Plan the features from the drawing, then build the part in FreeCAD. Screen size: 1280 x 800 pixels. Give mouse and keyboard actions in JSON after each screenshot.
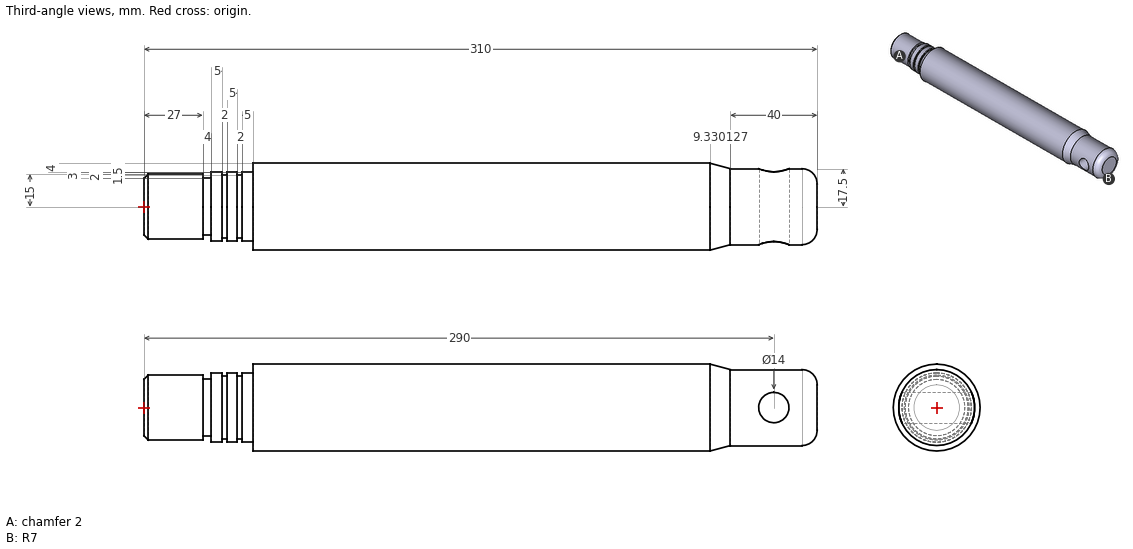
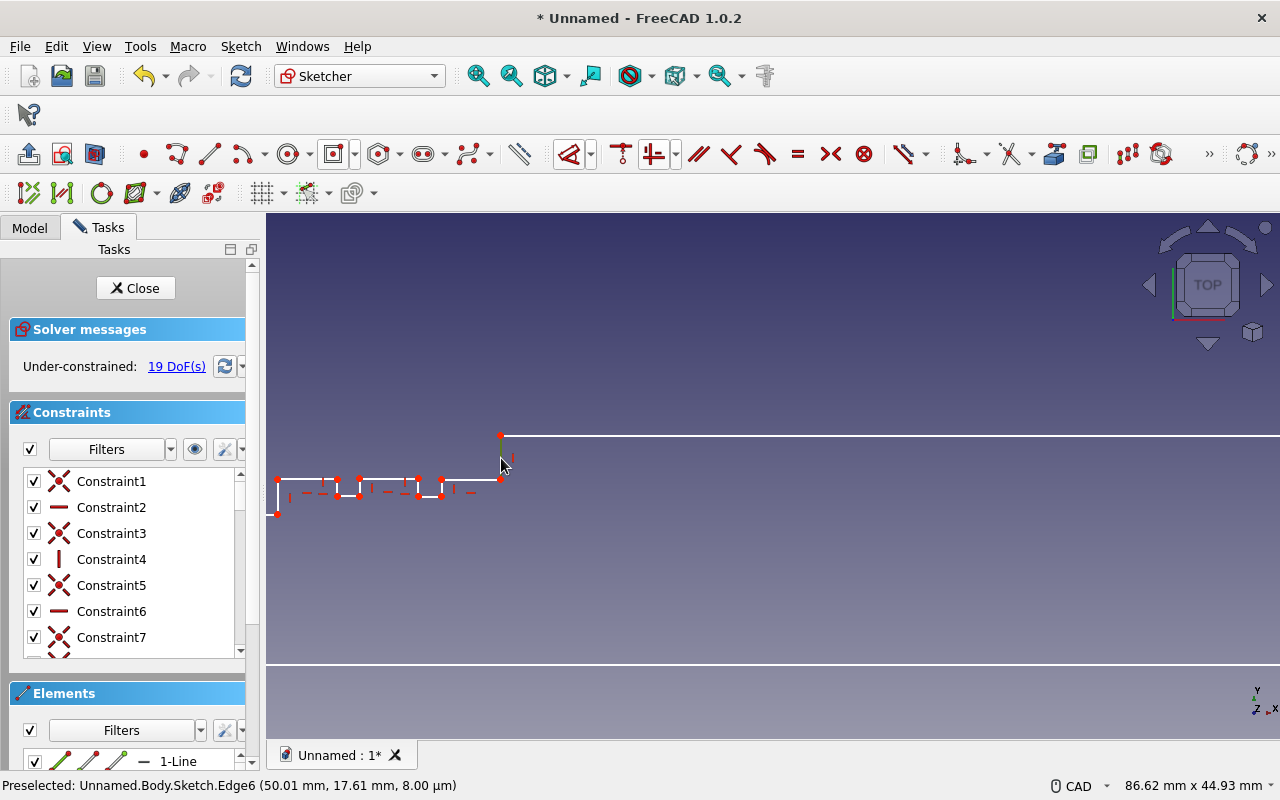
{"action": "left_click", "coordinate": [590, 154]}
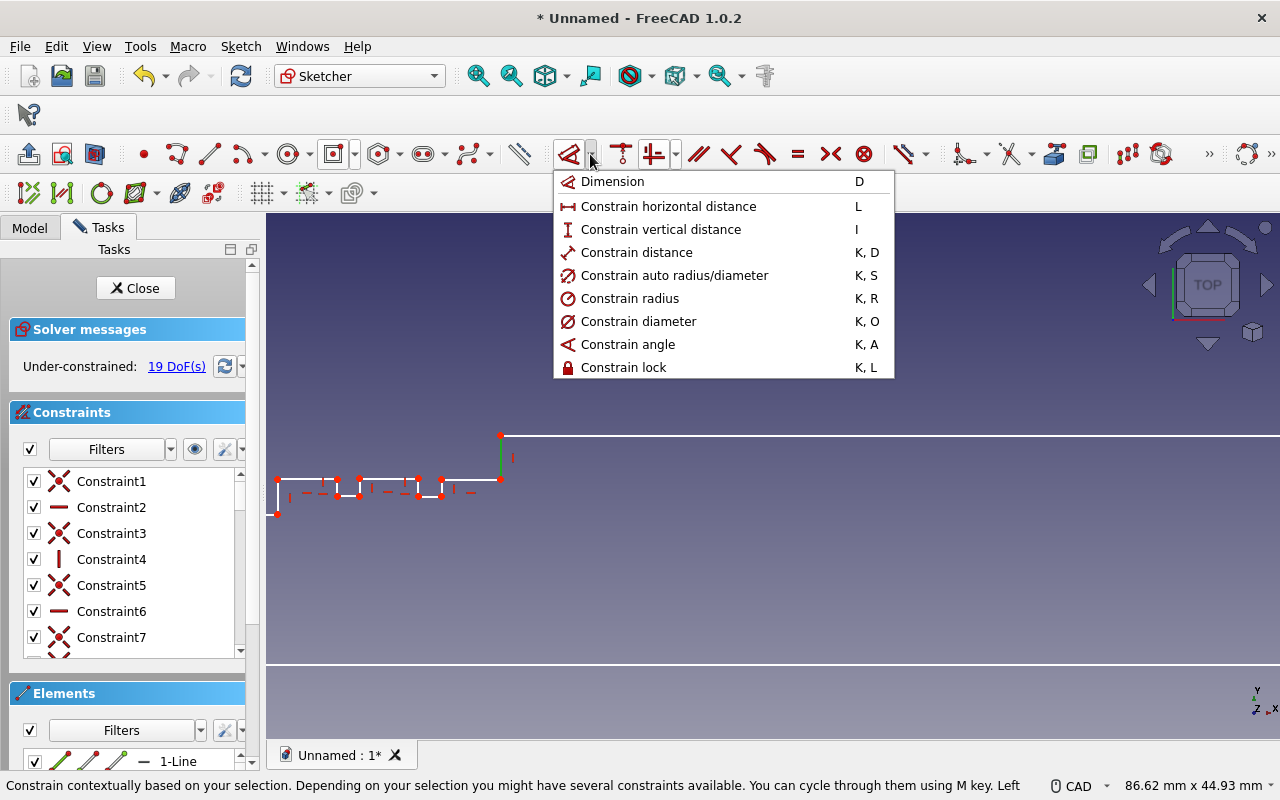
{"action": "left_click", "coordinate": [724, 230]}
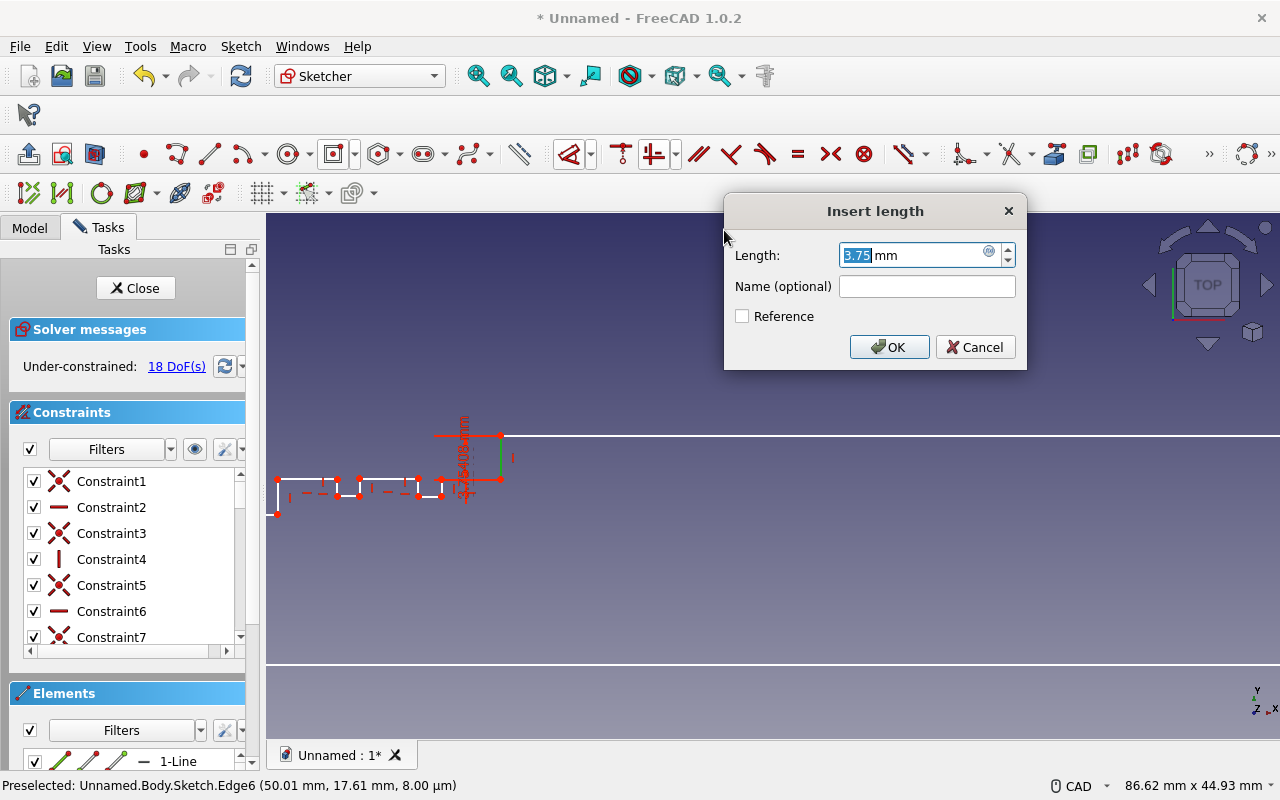
{"action": "type", "text": "4"}
{"action": "key", "text": "Return"}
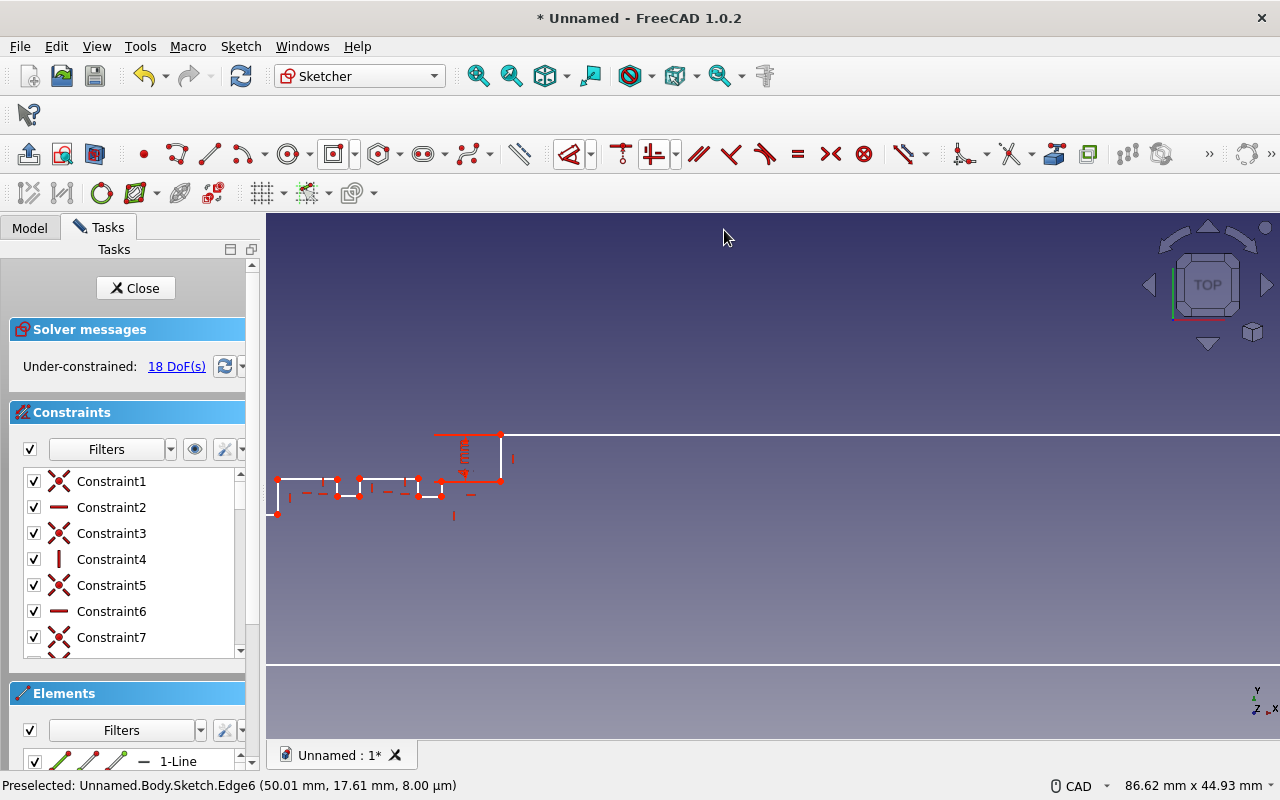
{"action": "left_click", "coordinate": [483, 482]}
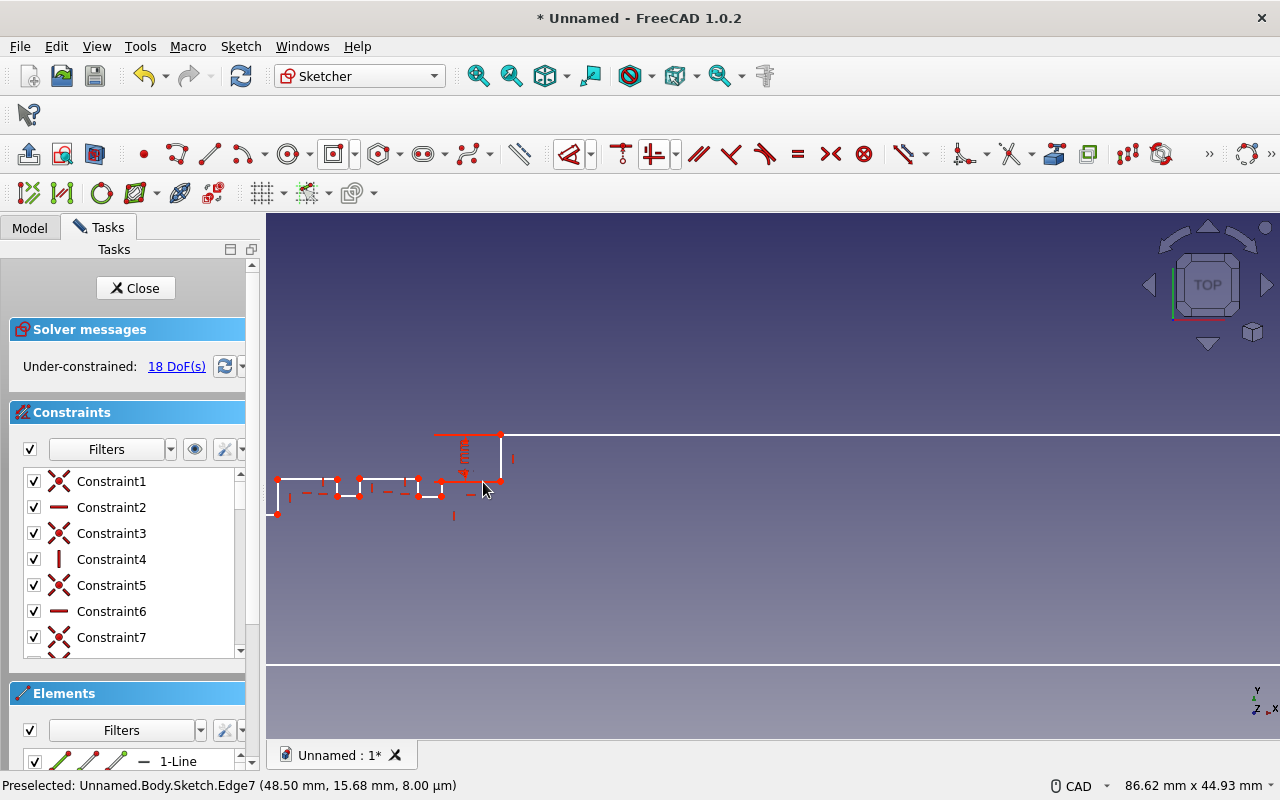
{"action": "key", "text": "l"}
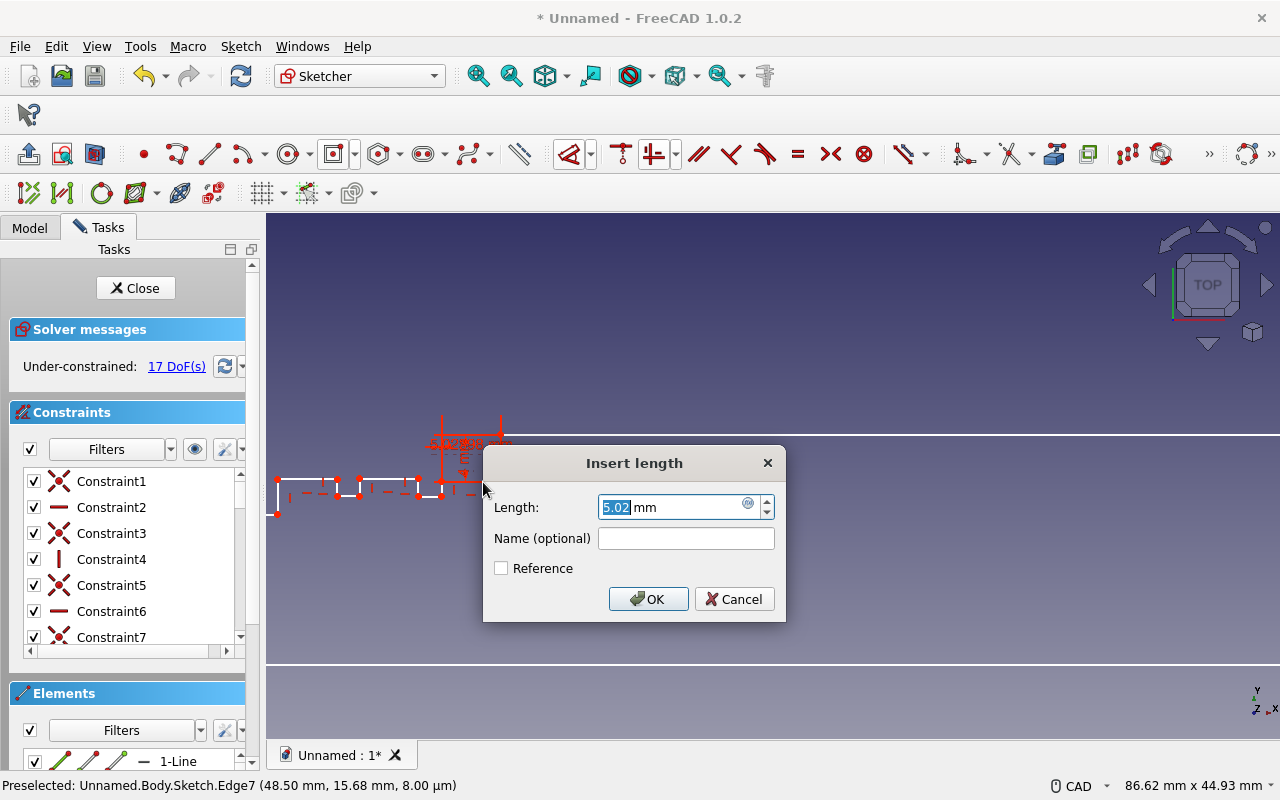
{"action": "type", "text": "5"}
{"action": "key", "text": "Return"}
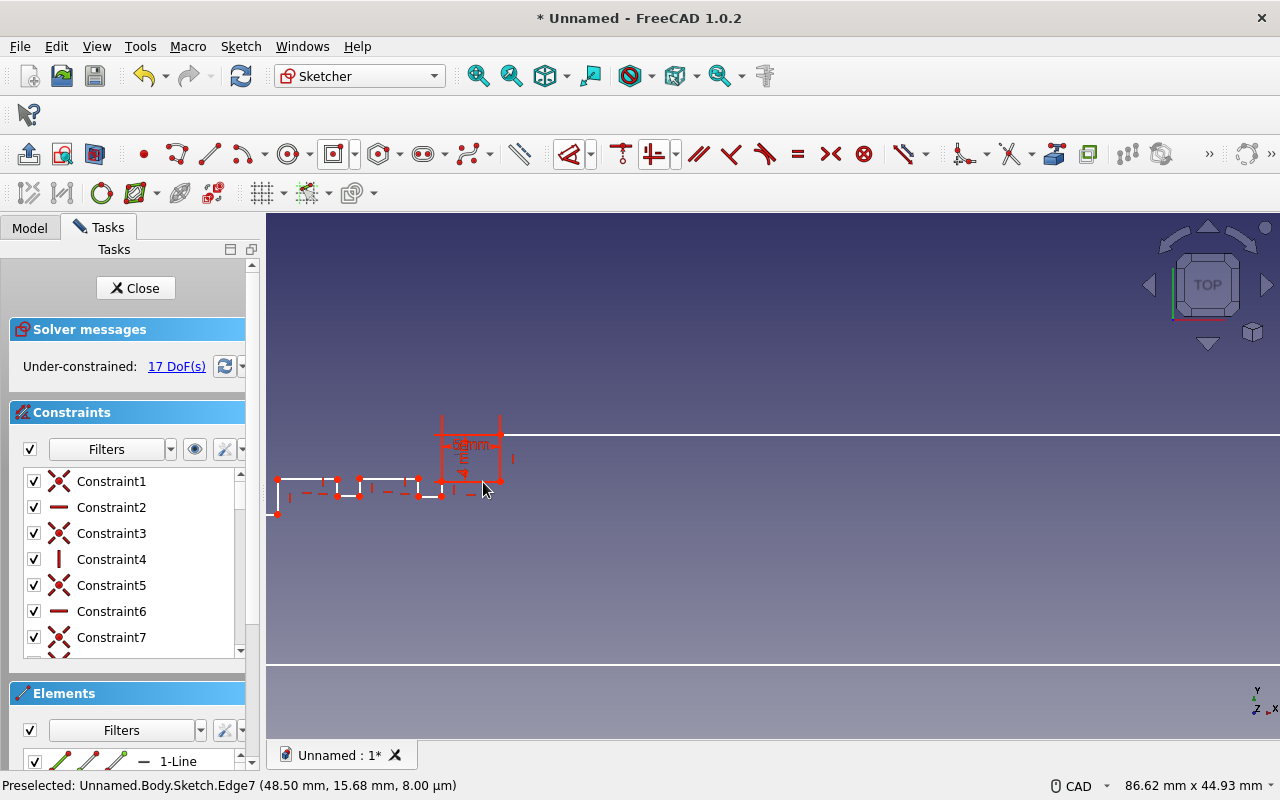
{"action": "scroll", "coordinate": [432, 497], "scroll_direction": "up", "scroll_amount": 3}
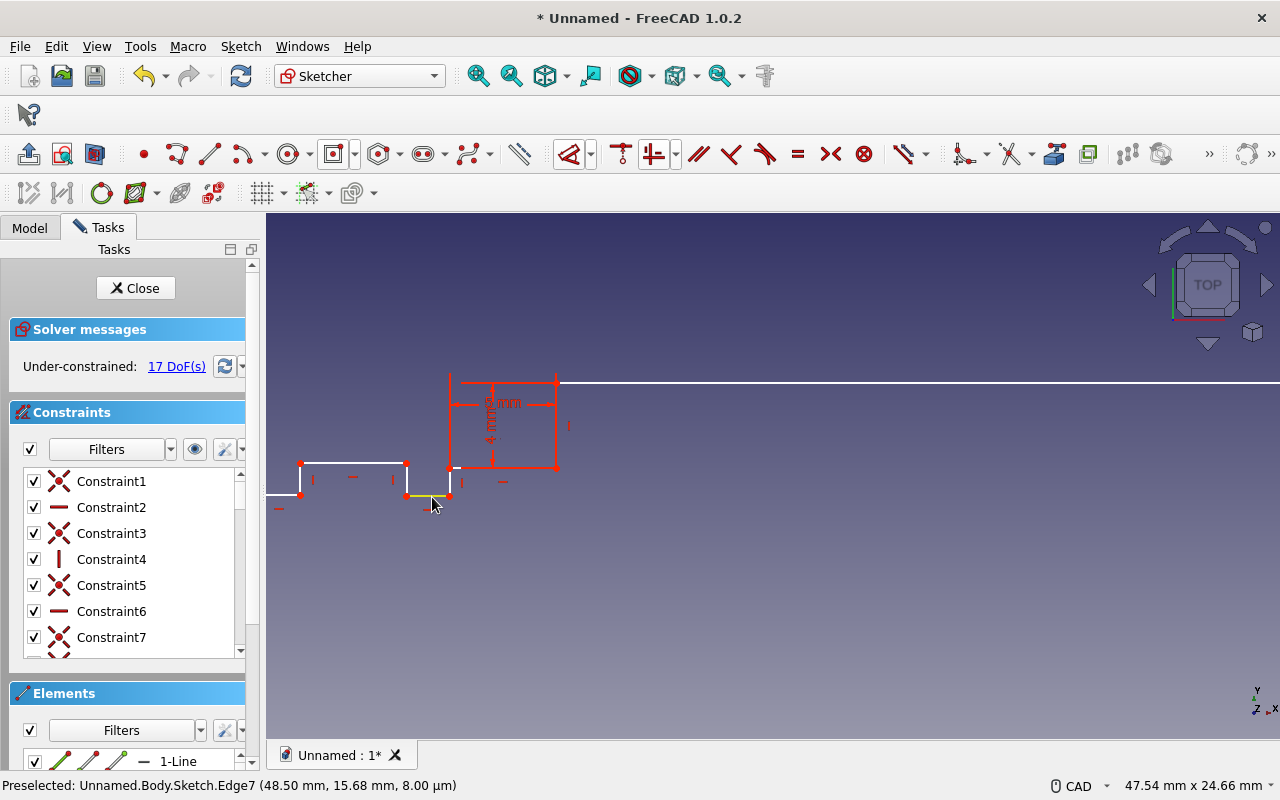
{"action": "left_click", "coordinate": [433, 496]}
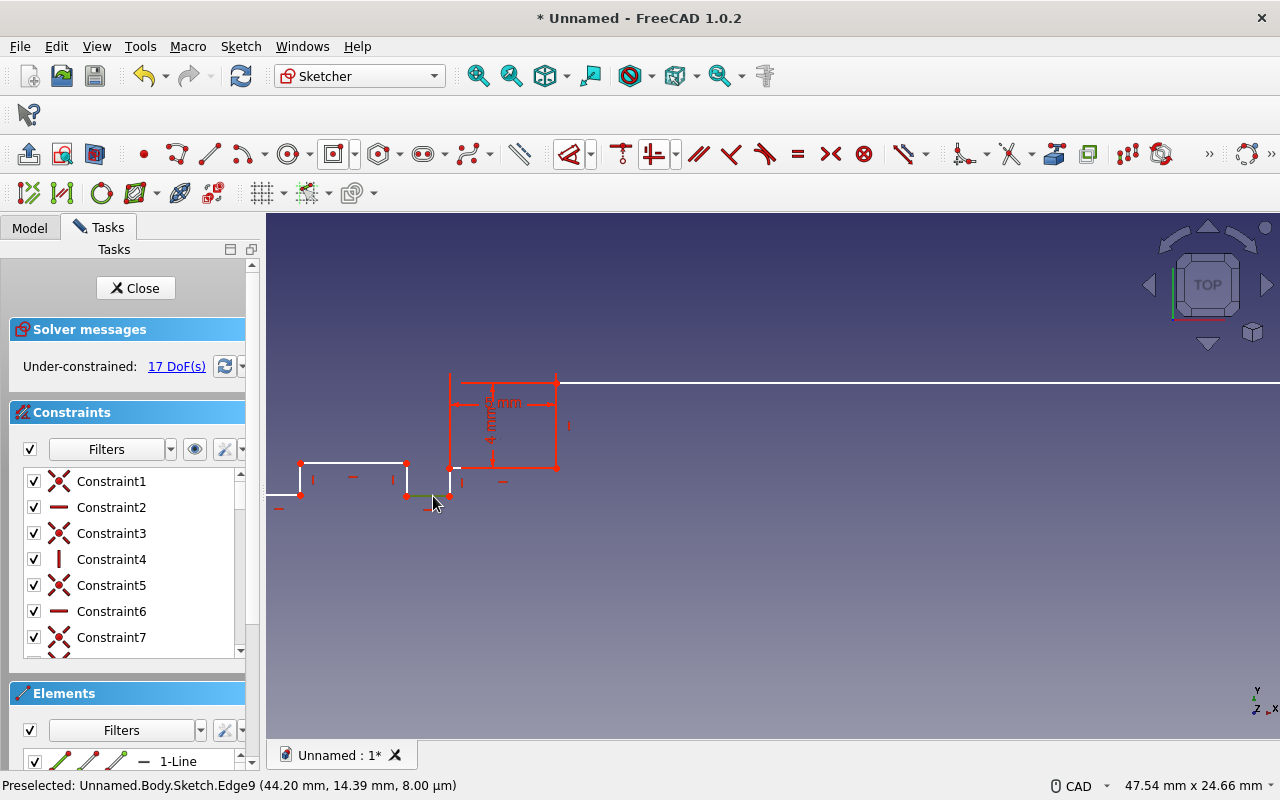
{"action": "left_click", "coordinate": [590, 154]}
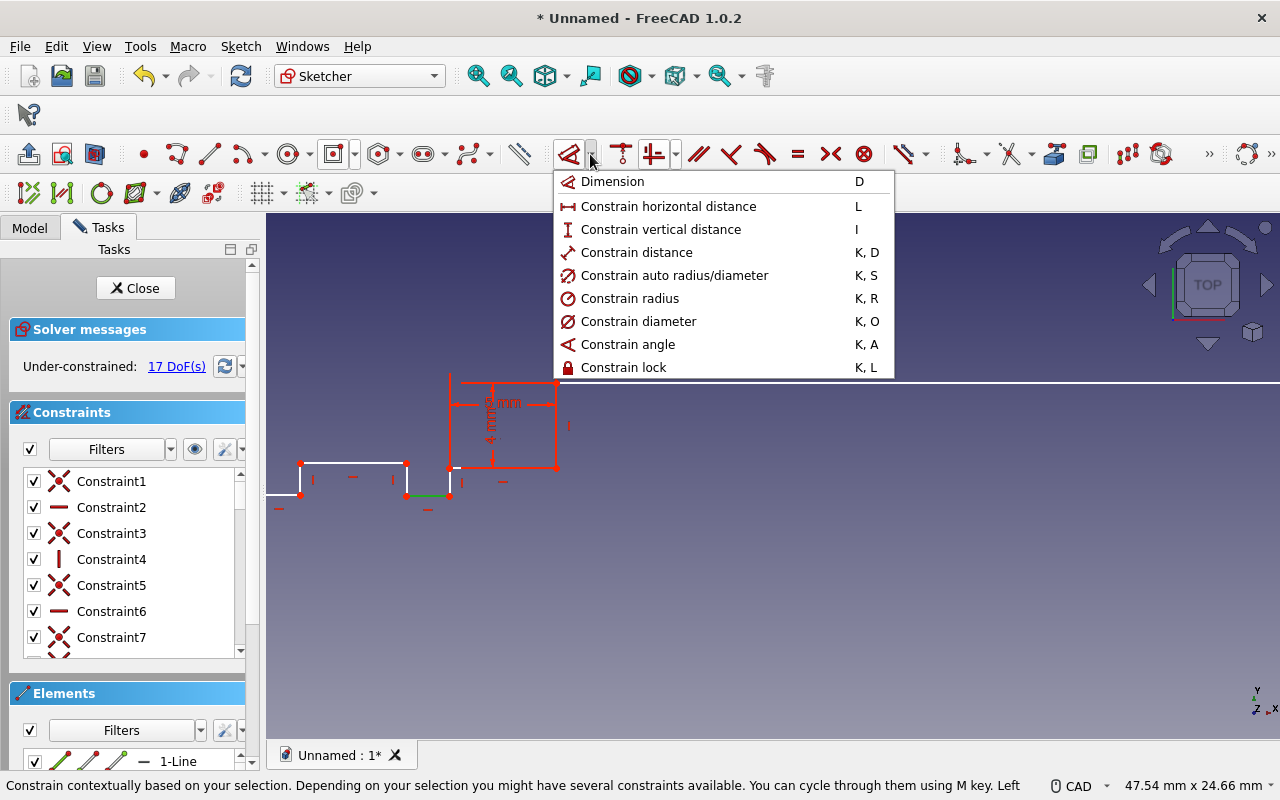
{"action": "left_click", "coordinate": [724, 206]}